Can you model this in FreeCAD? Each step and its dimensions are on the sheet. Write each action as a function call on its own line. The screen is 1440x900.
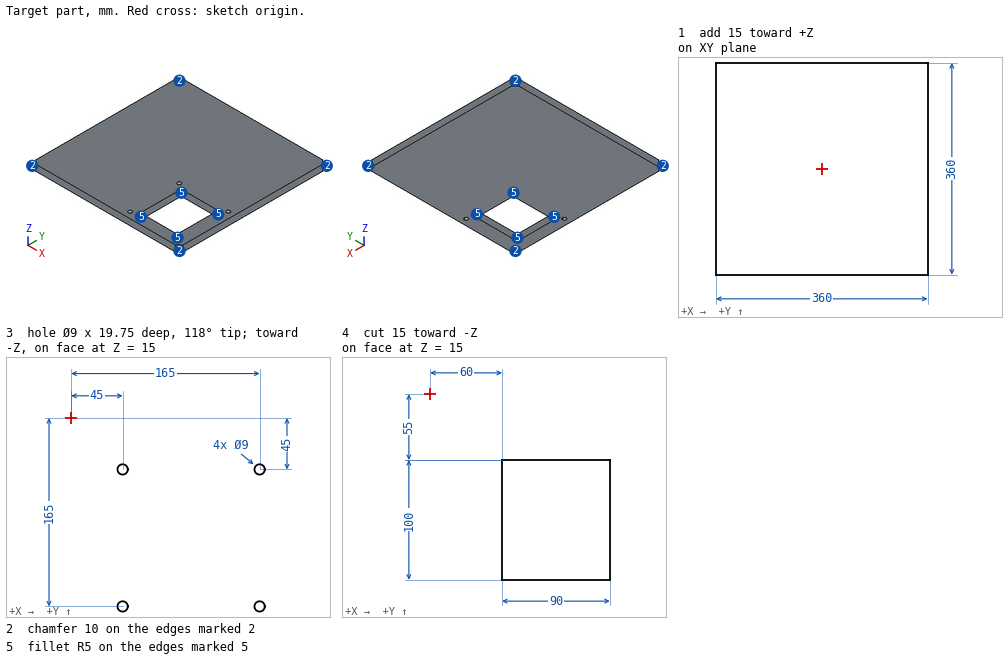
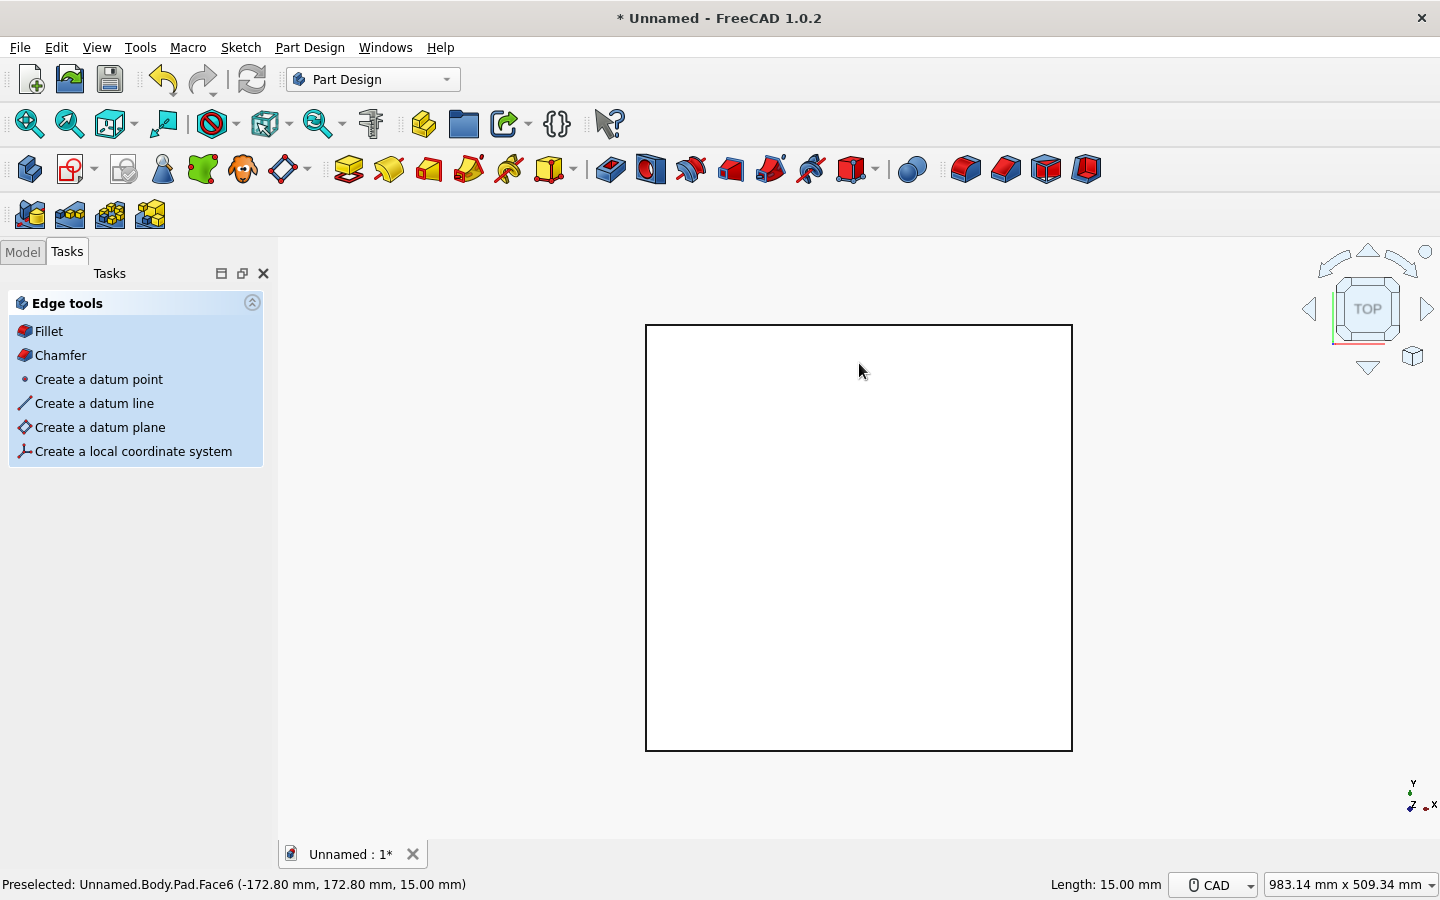
scroll(646, 324, up, 5)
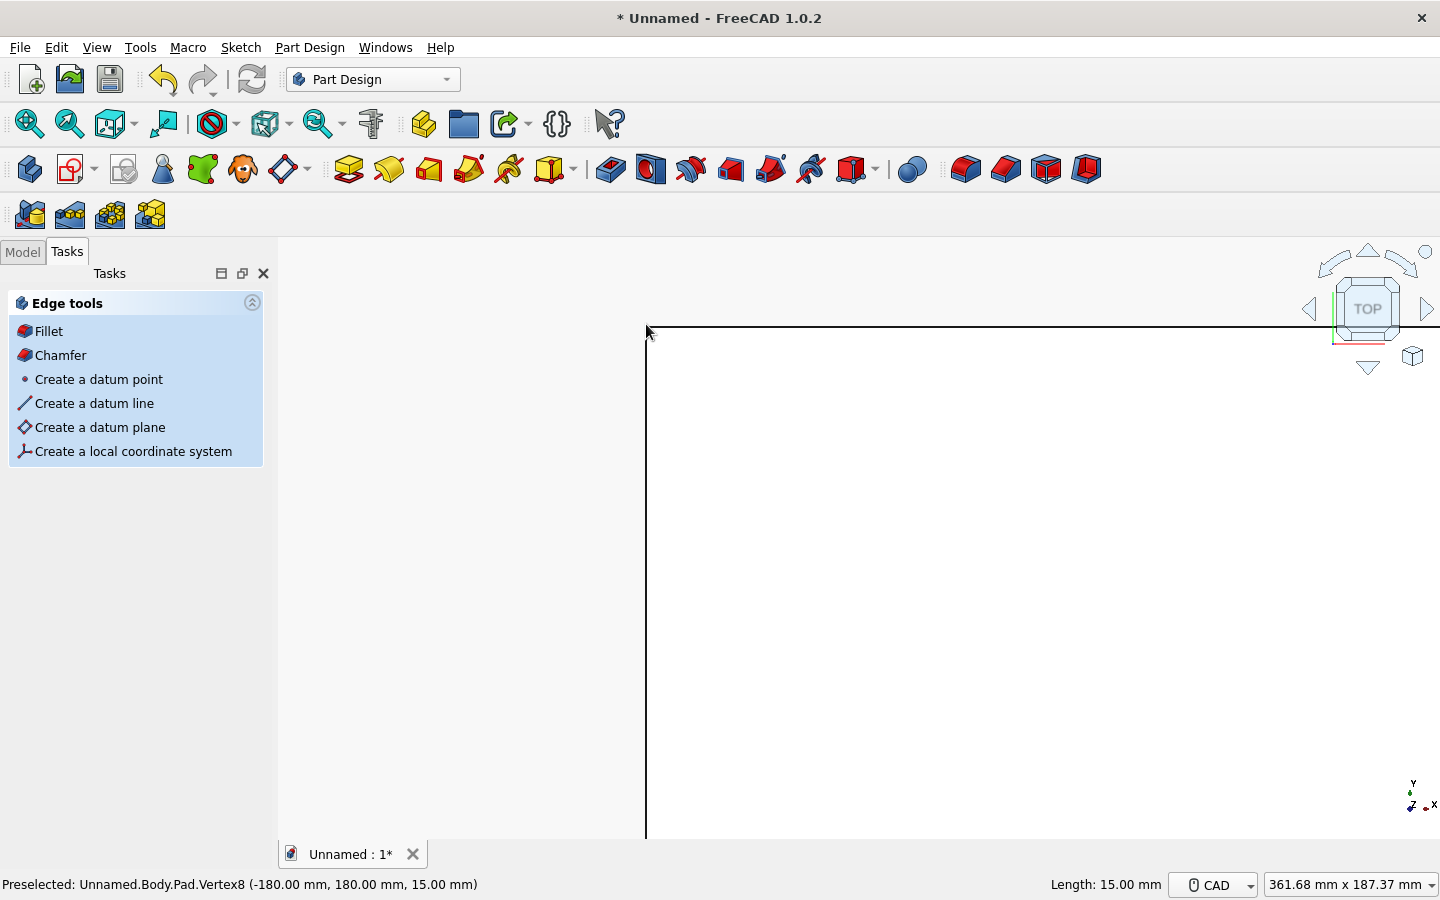
key(v)
key(f)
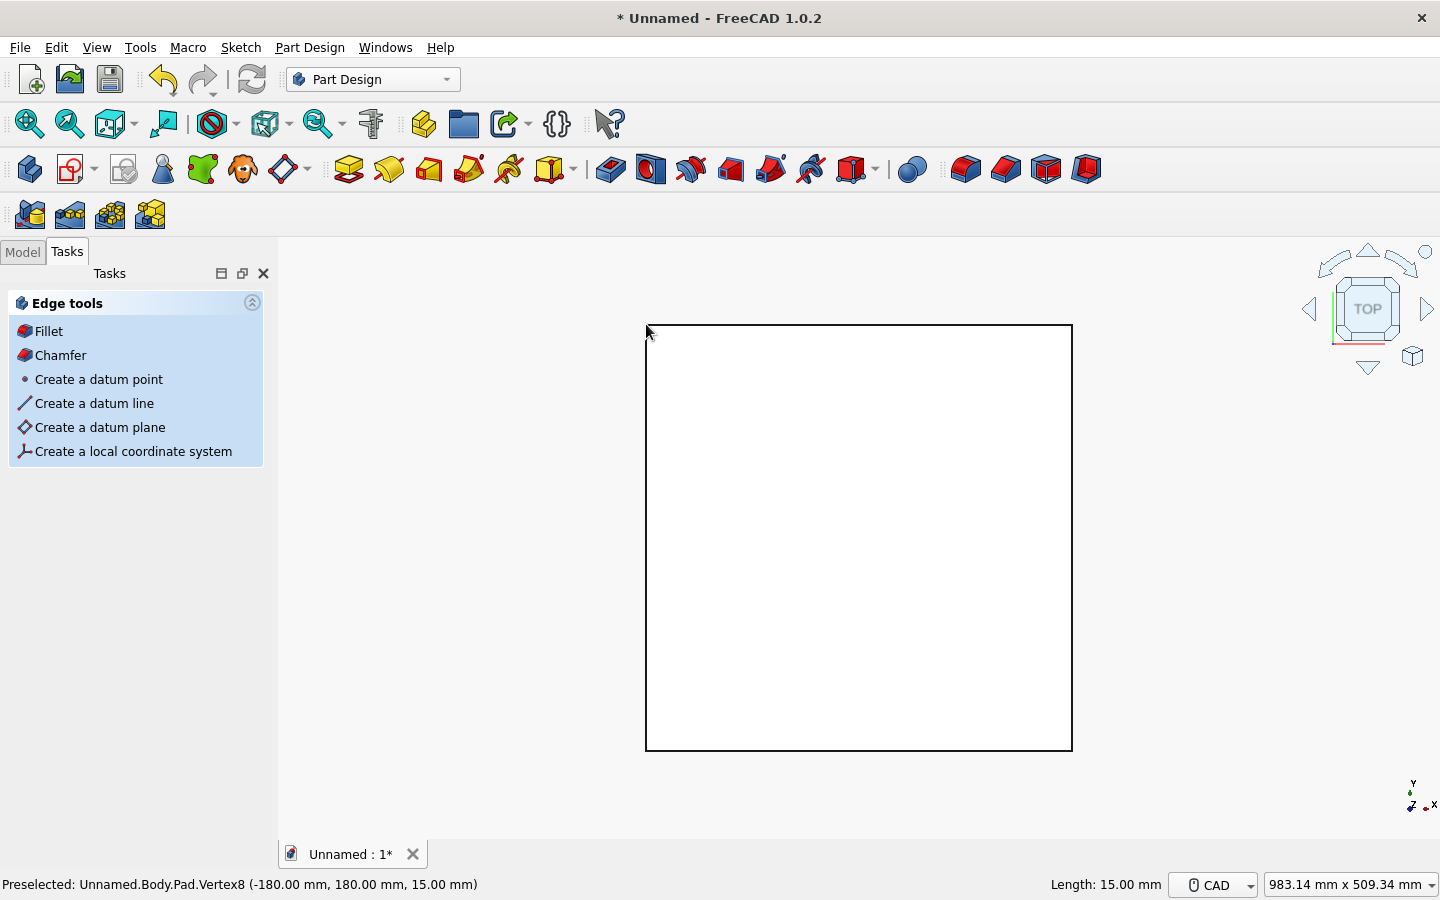
key(1)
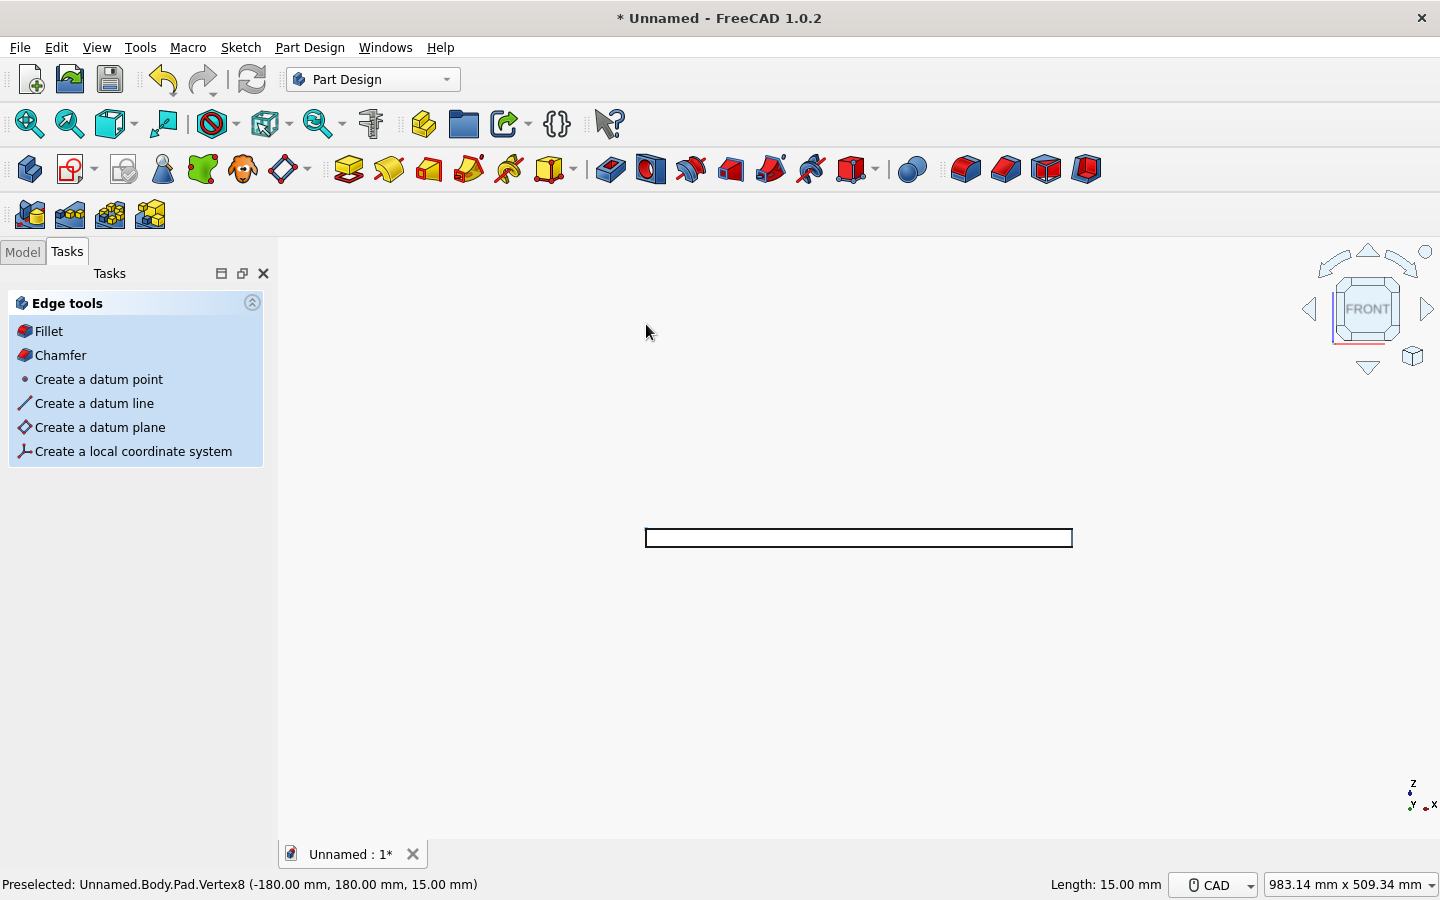
key(v)
key(f)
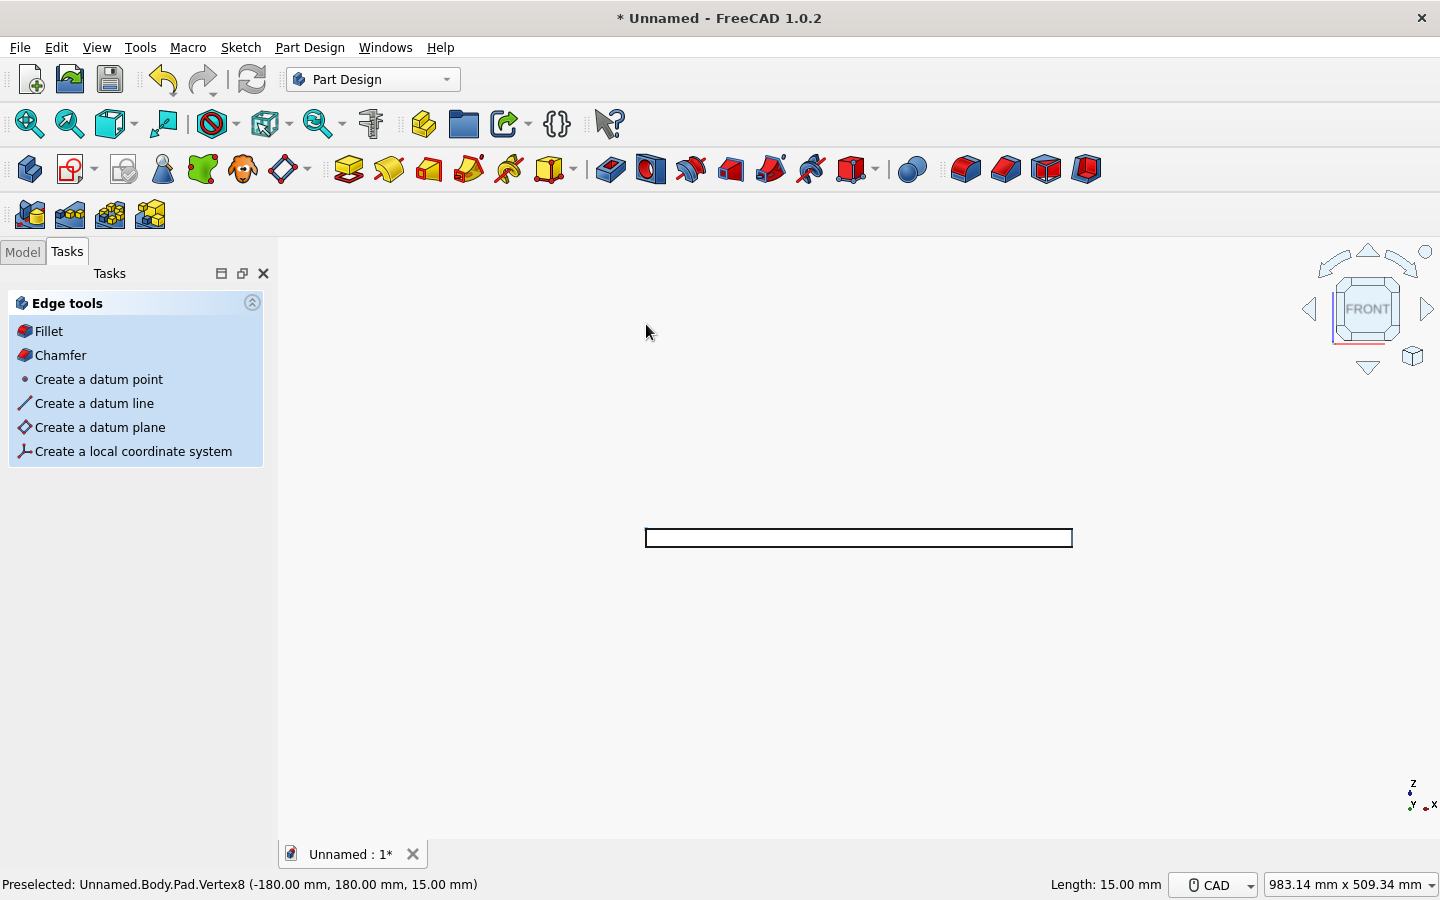
click(646, 537, ctrl)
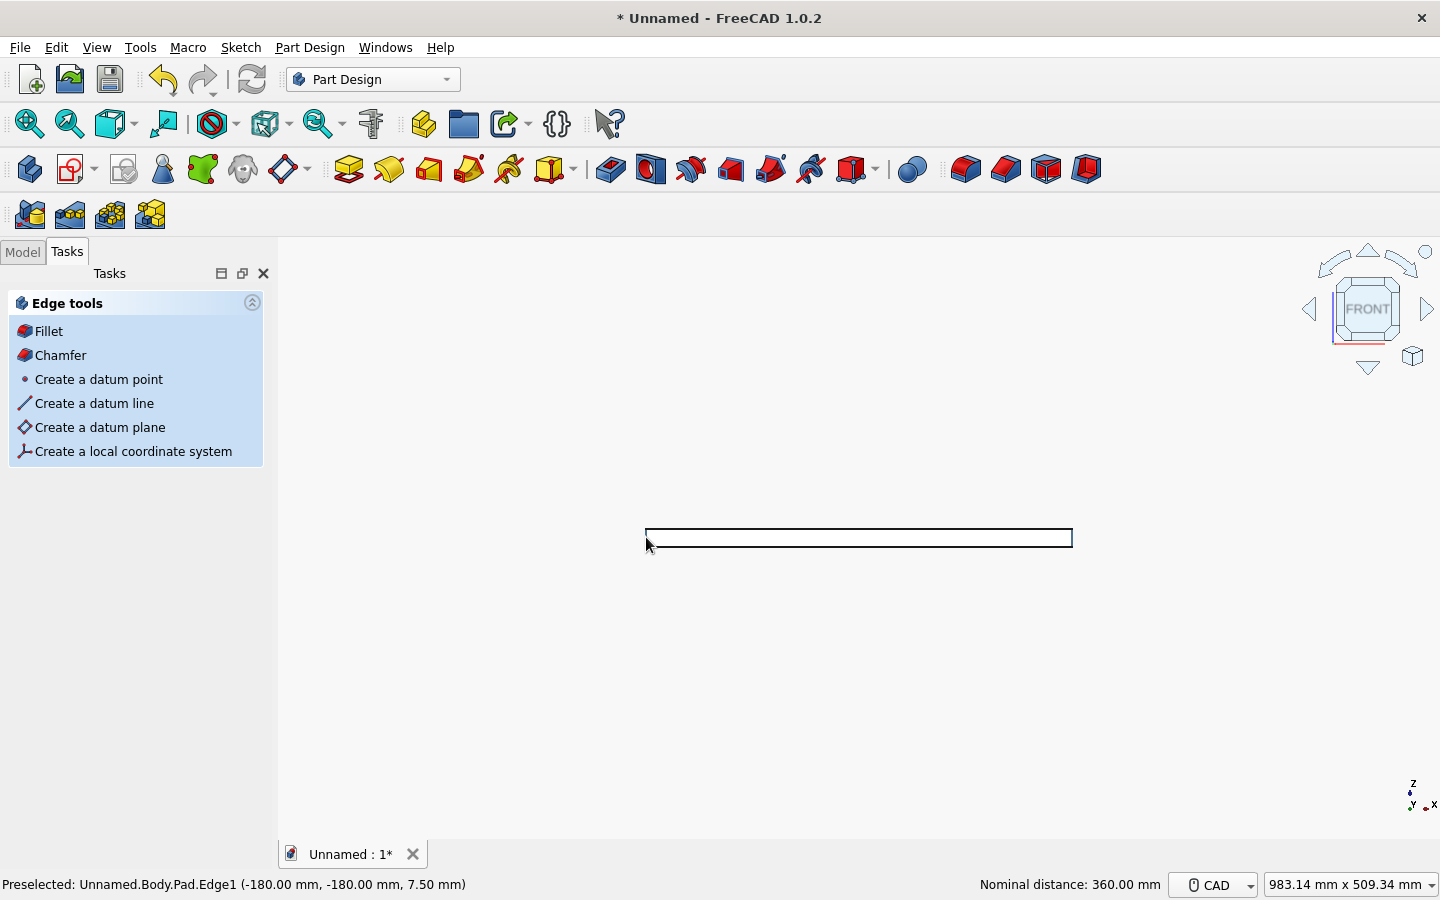
scroll(646, 537, up, 5)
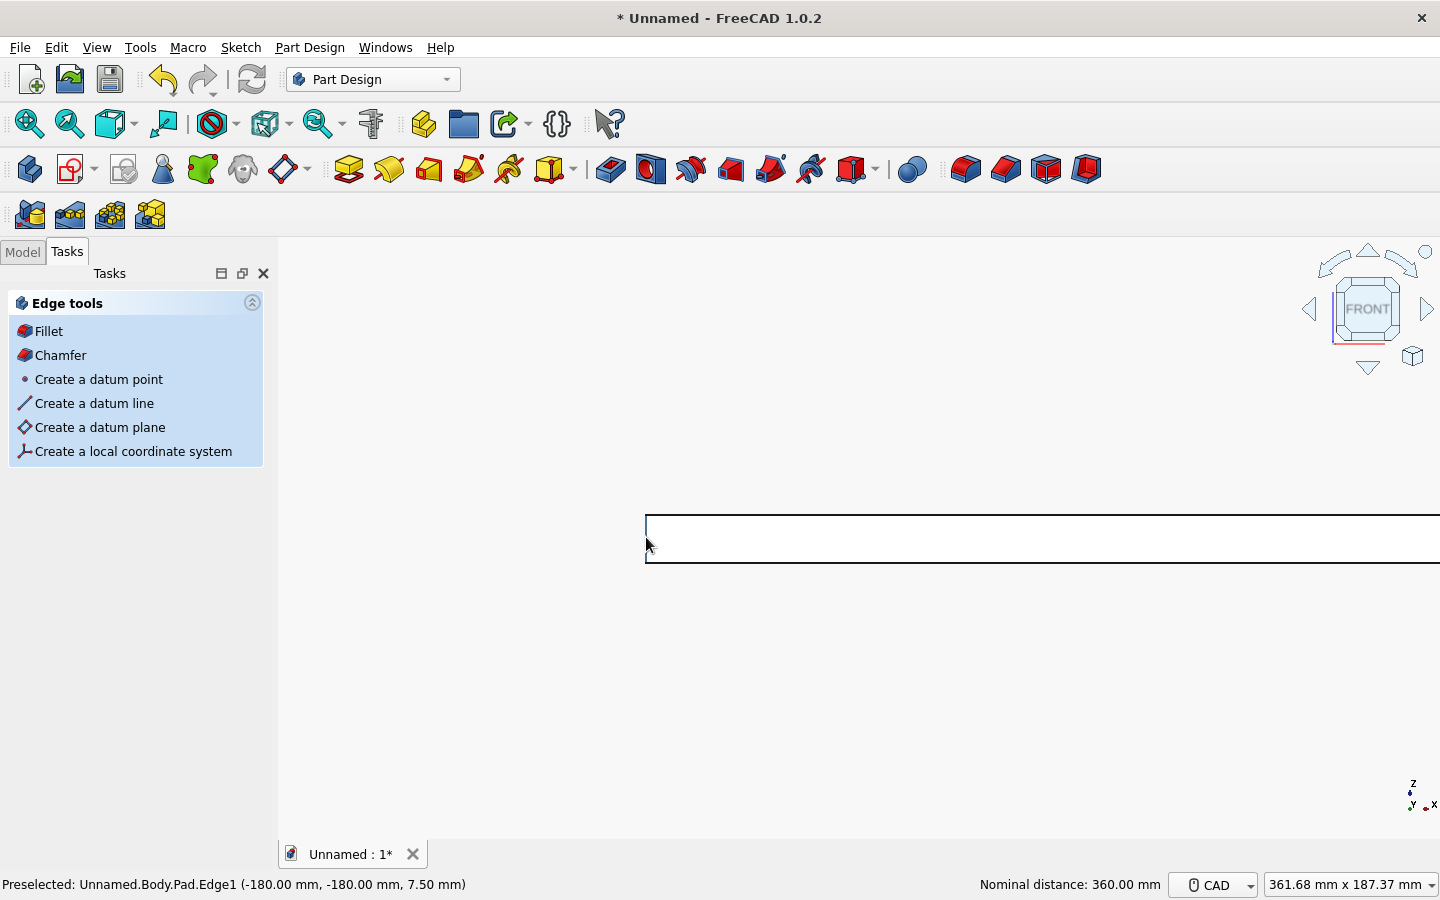
click(30, 124)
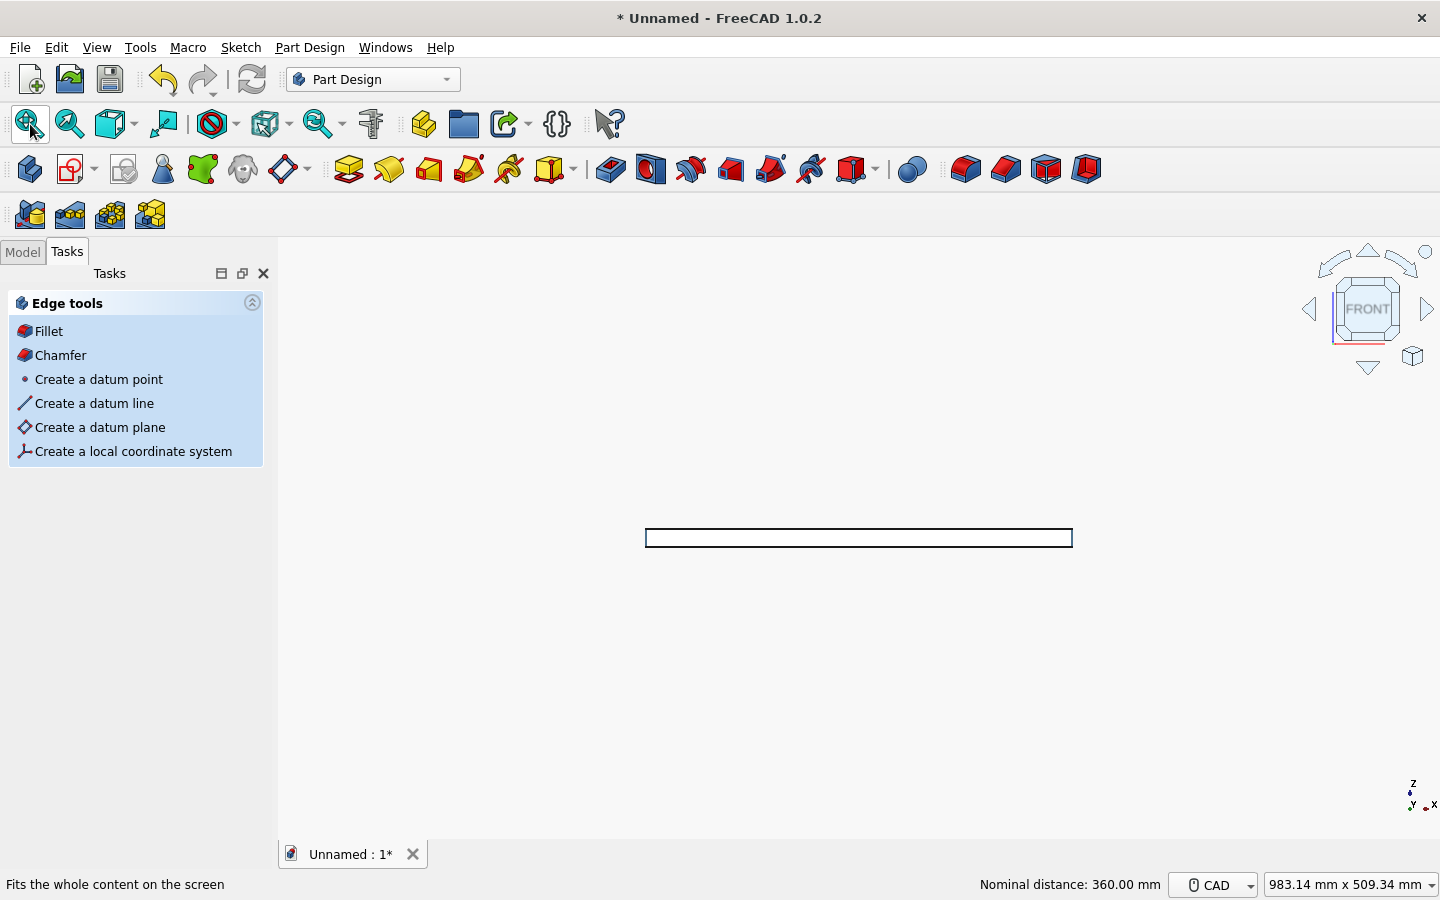
key(3)